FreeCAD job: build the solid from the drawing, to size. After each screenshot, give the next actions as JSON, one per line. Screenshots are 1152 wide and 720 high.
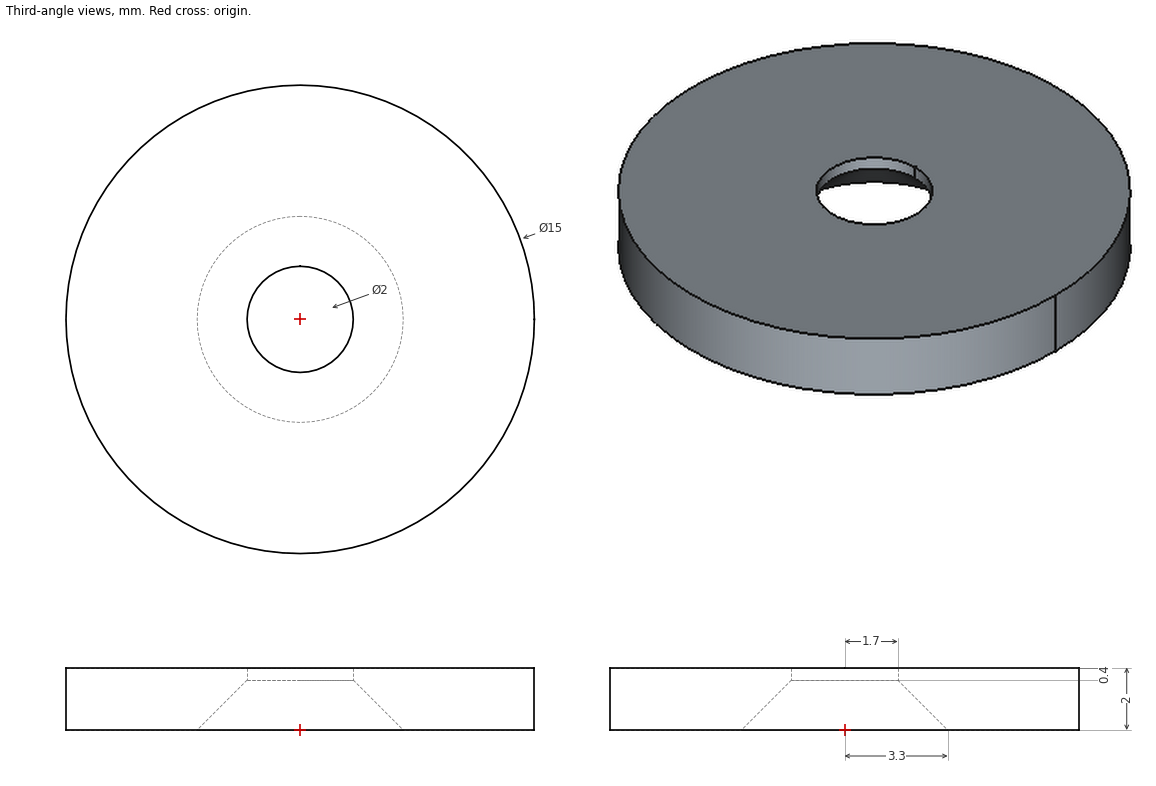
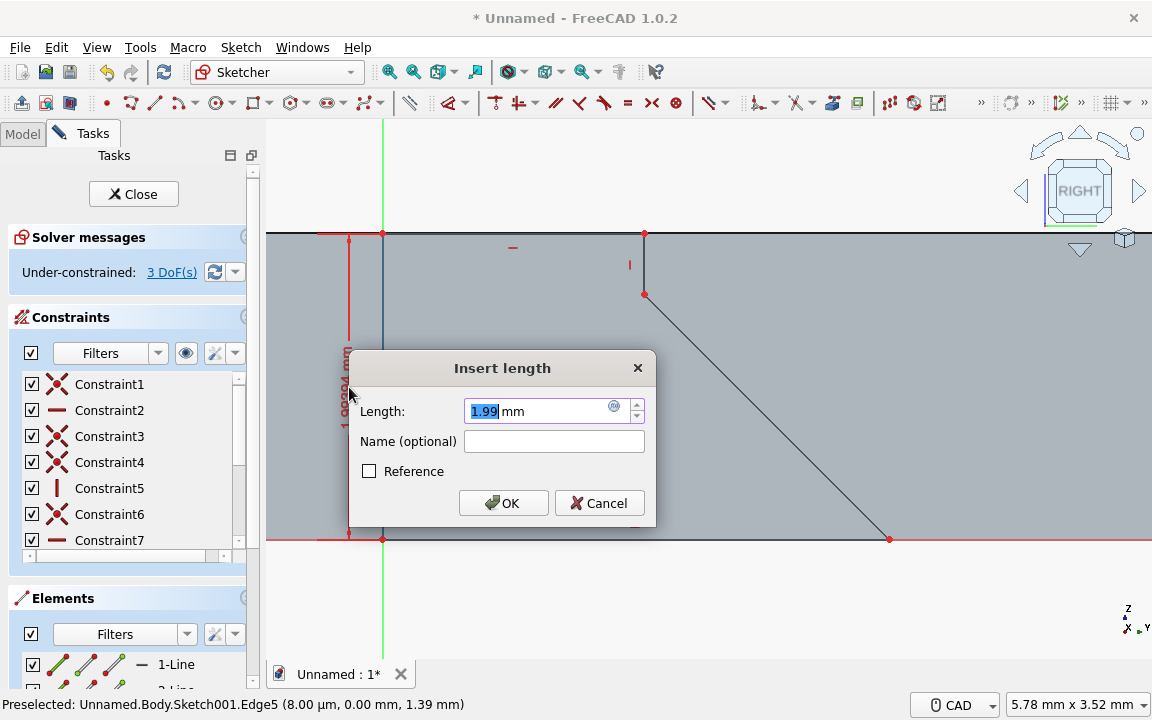
{"action": "type", "text": "2"}
{"action": "key", "text": "Return"}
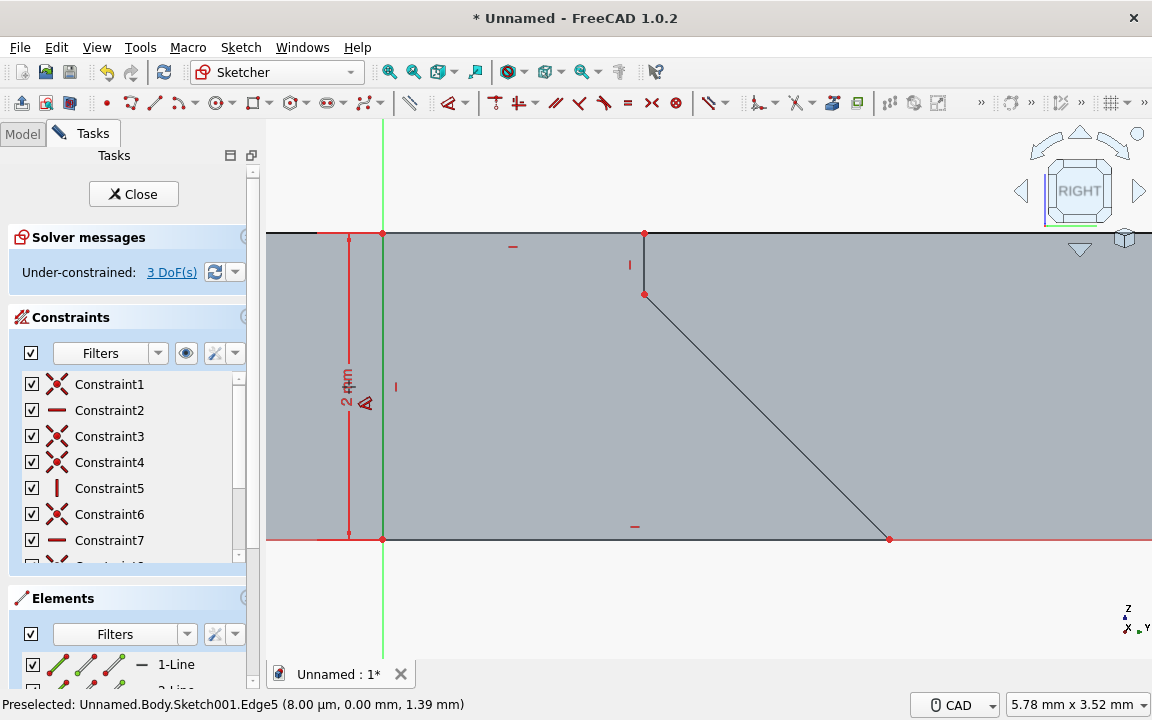
{"action": "left_click", "coordinate": [535, 540]}
{"action": "left_click", "coordinate": [636, 574]}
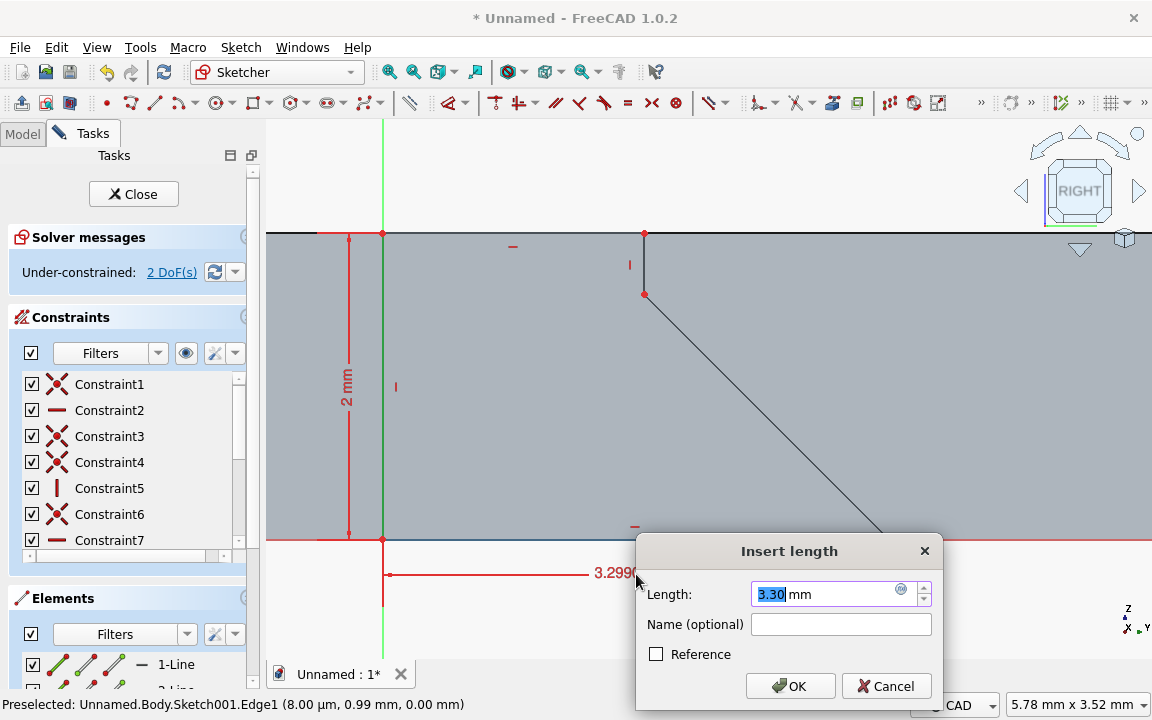
{"action": "type", "text": "3.3"}
{"action": "key", "text": "Return"}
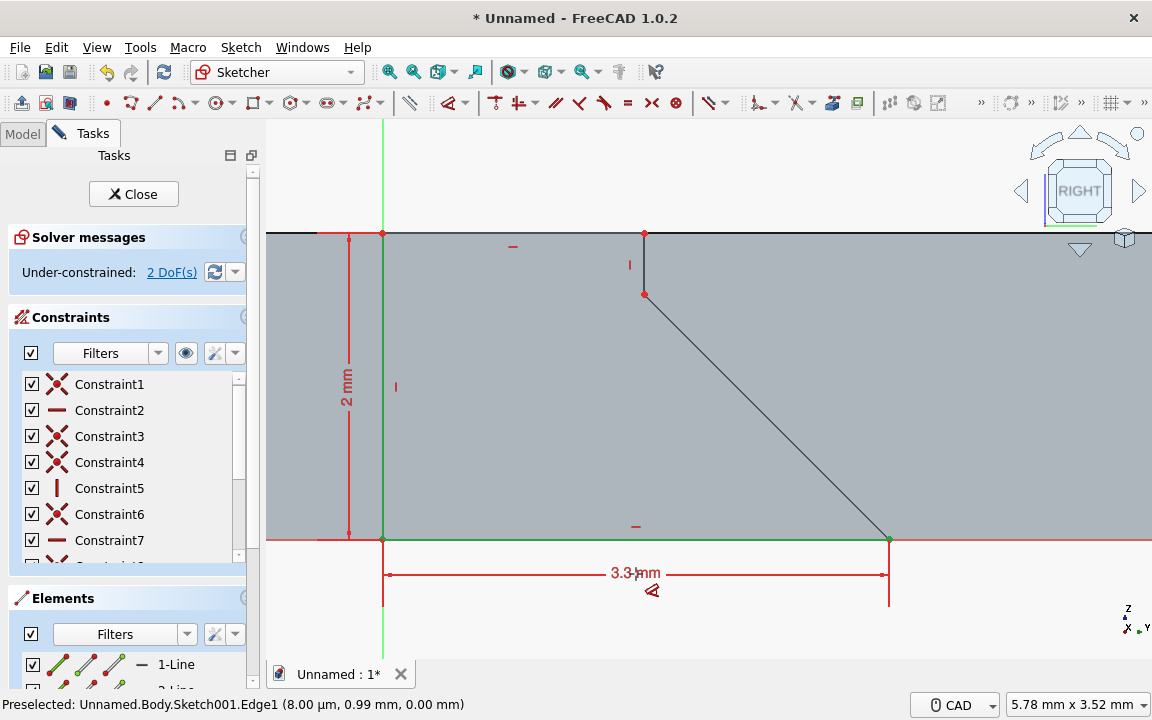
{"action": "left_click", "coordinate": [644, 276]}
{"action": "left_click", "coordinate": [678, 264]}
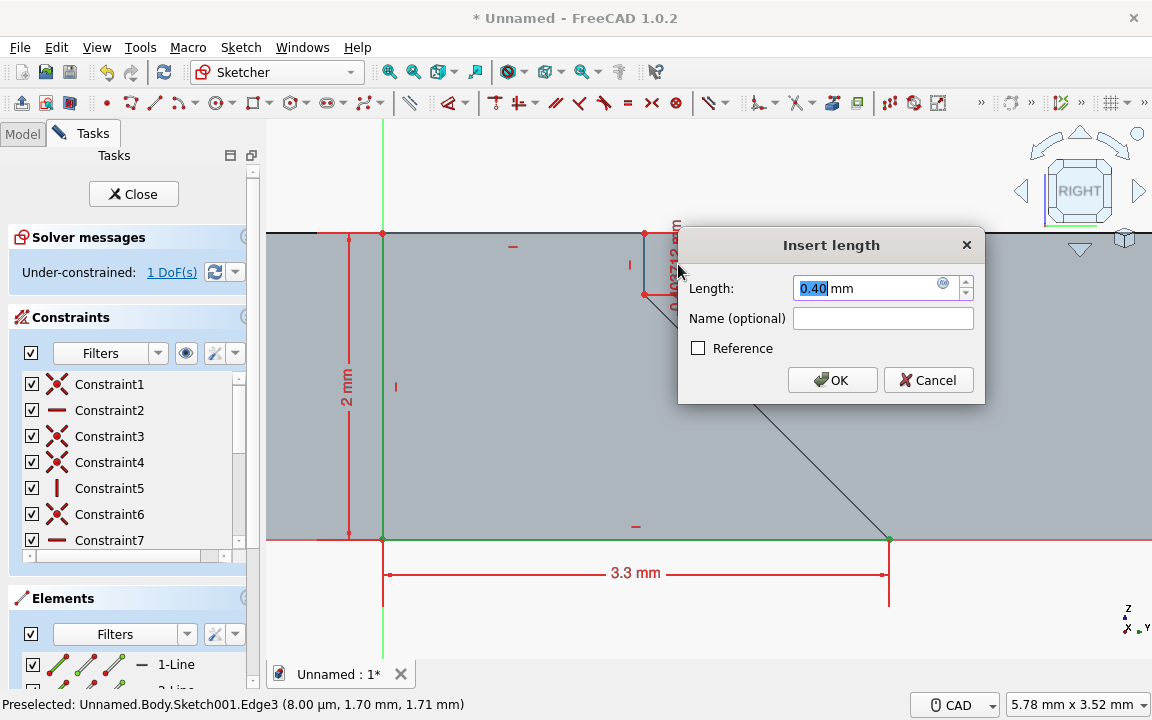
{"action": "type", "text": "0.4"}
{"action": "key", "text": "Return"}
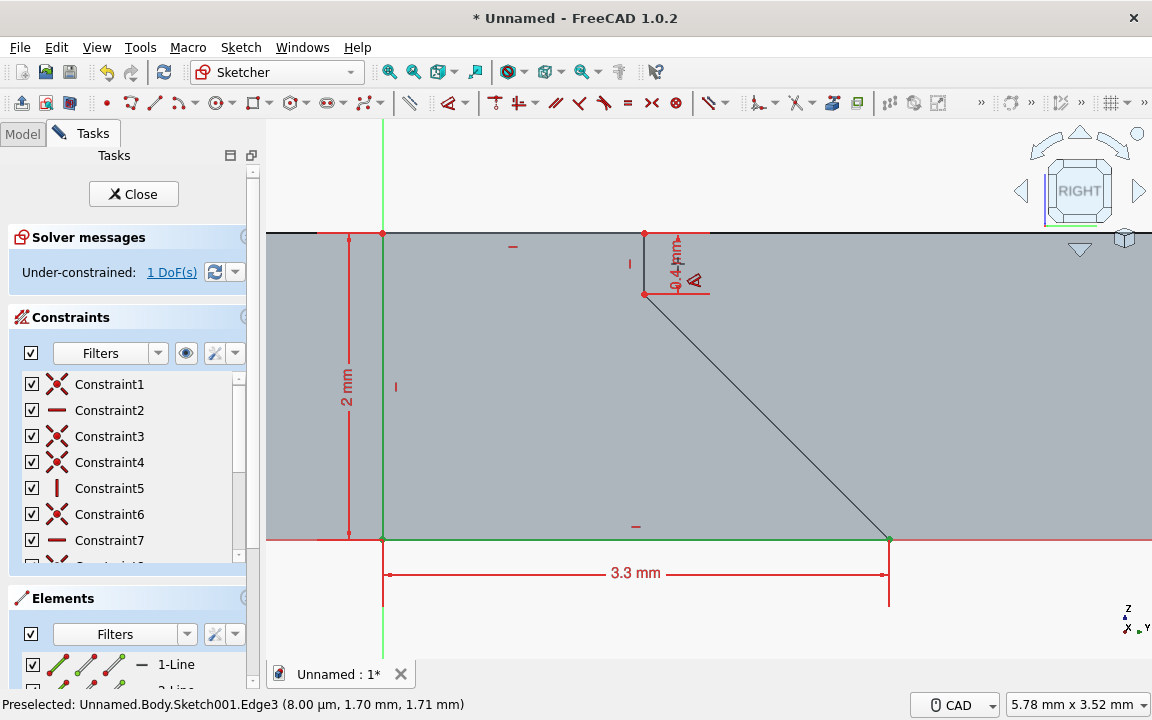
{"action": "left_click", "coordinate": [566, 233]}
{"action": "left_click", "coordinate": [513, 199]}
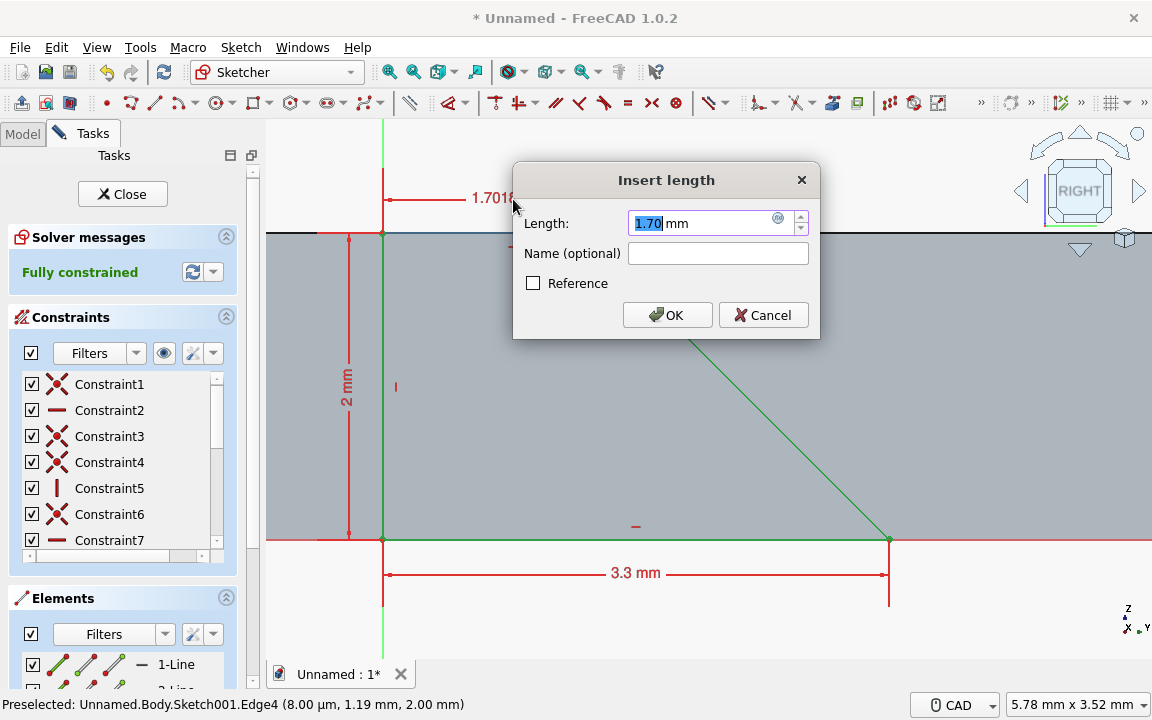
{"action": "type", "text": "1.7"}
{"action": "key", "text": "Return"}
{"action": "key", "text": "Escape"}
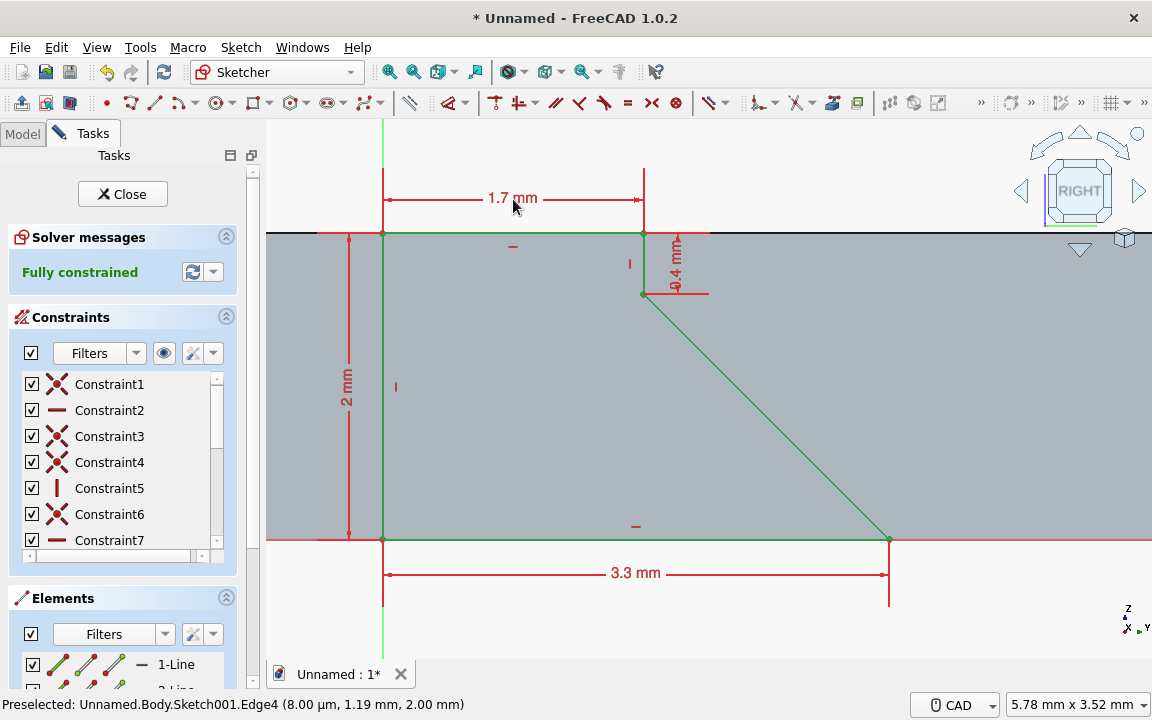
{"action": "left_click", "coordinate": [123, 194]}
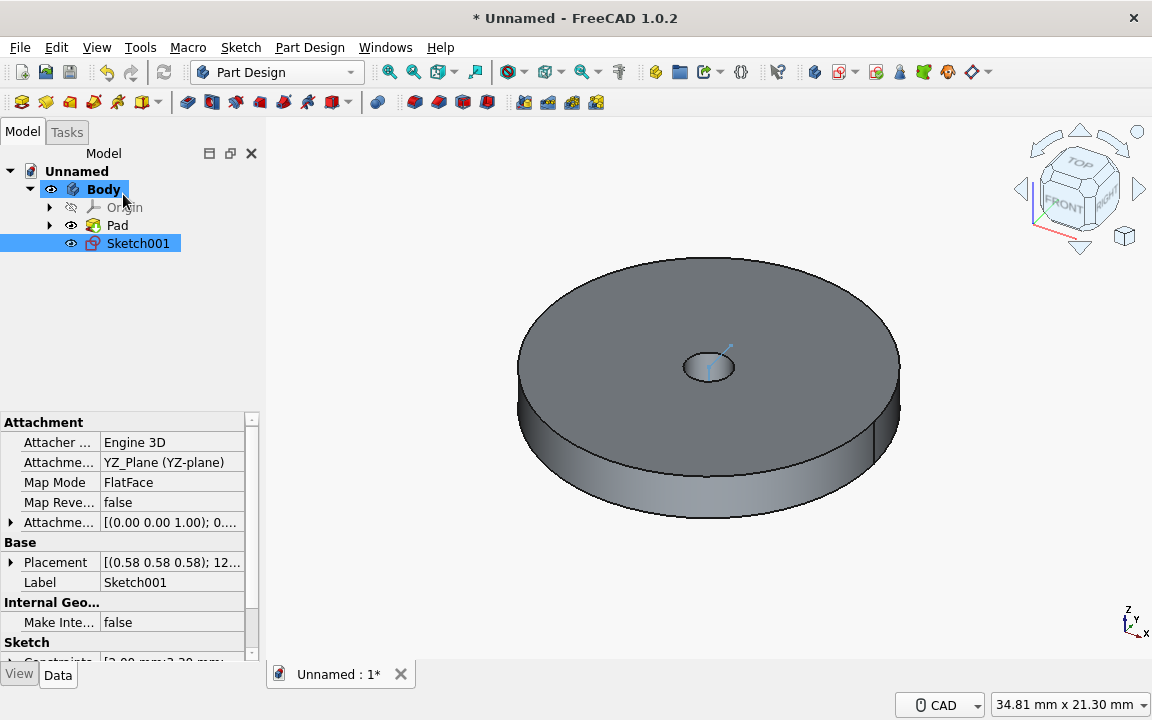
{"action": "left_click", "coordinate": [236, 102]}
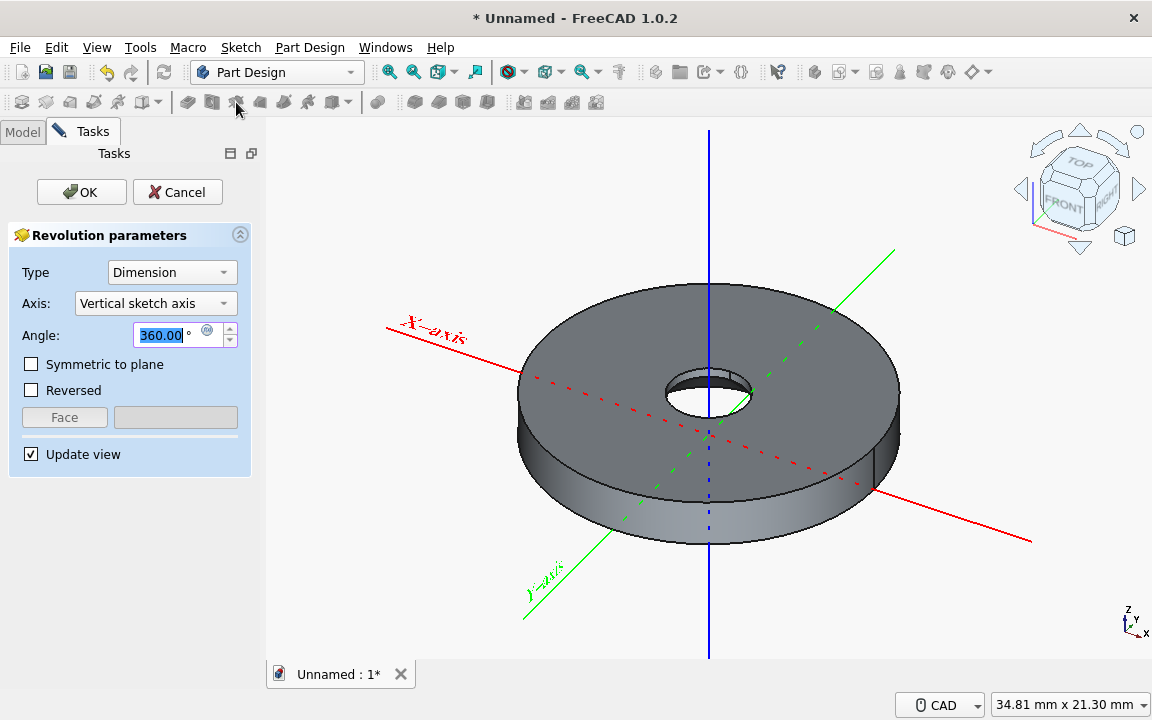
{"action": "left_click", "coordinate": [82, 192]}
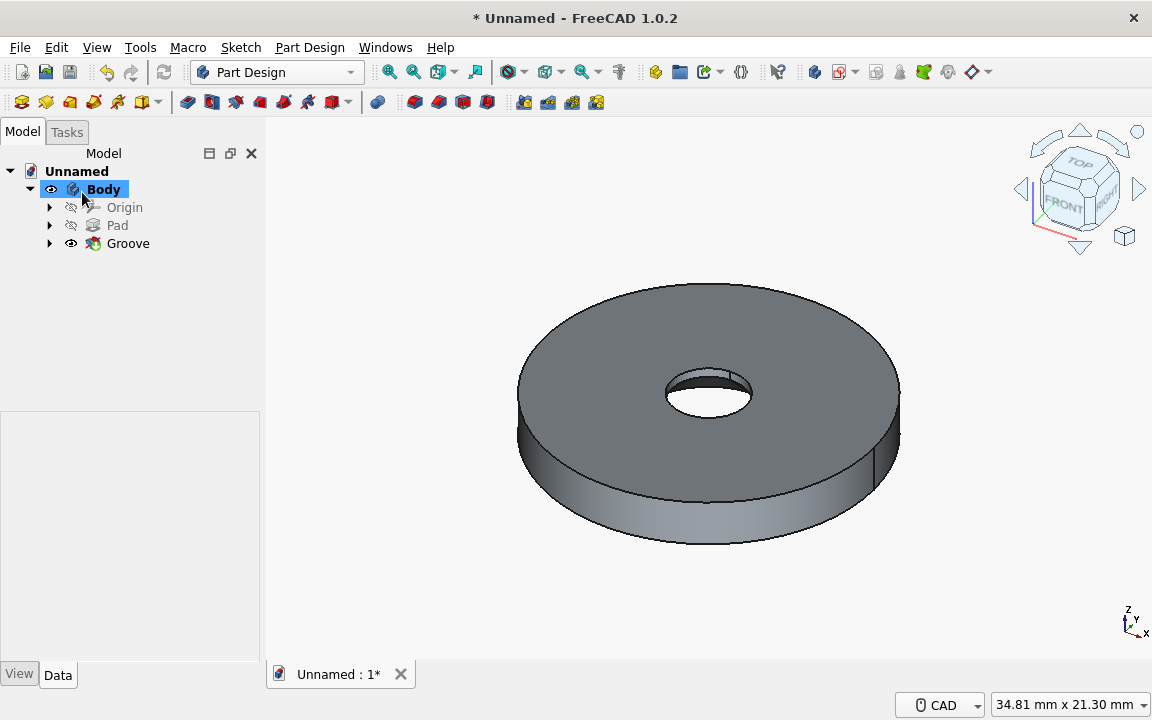
{"action": "key", "text": "0"}